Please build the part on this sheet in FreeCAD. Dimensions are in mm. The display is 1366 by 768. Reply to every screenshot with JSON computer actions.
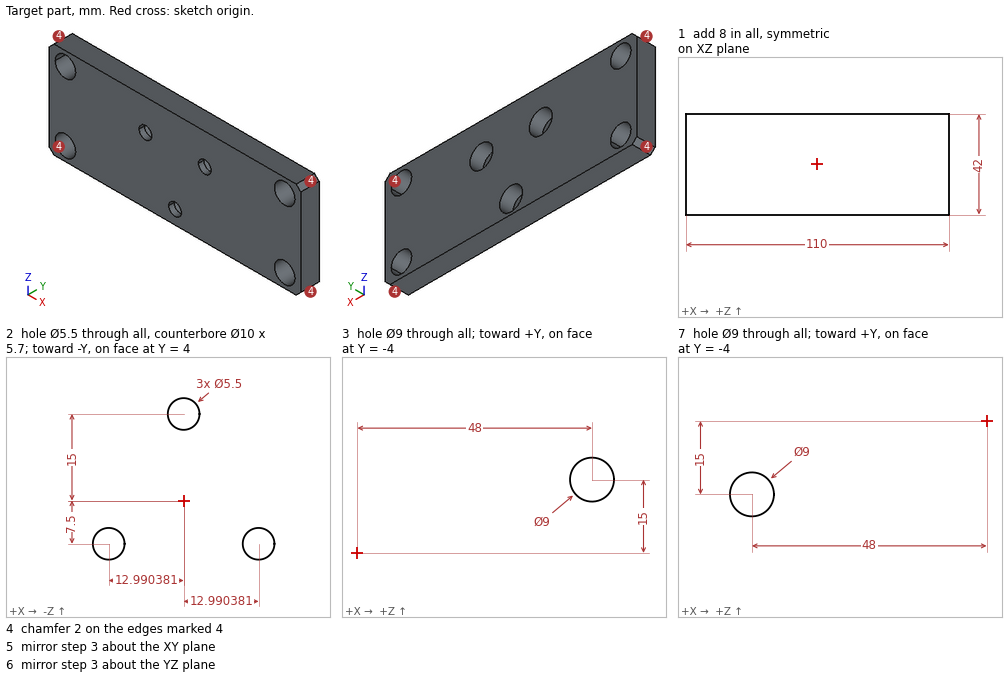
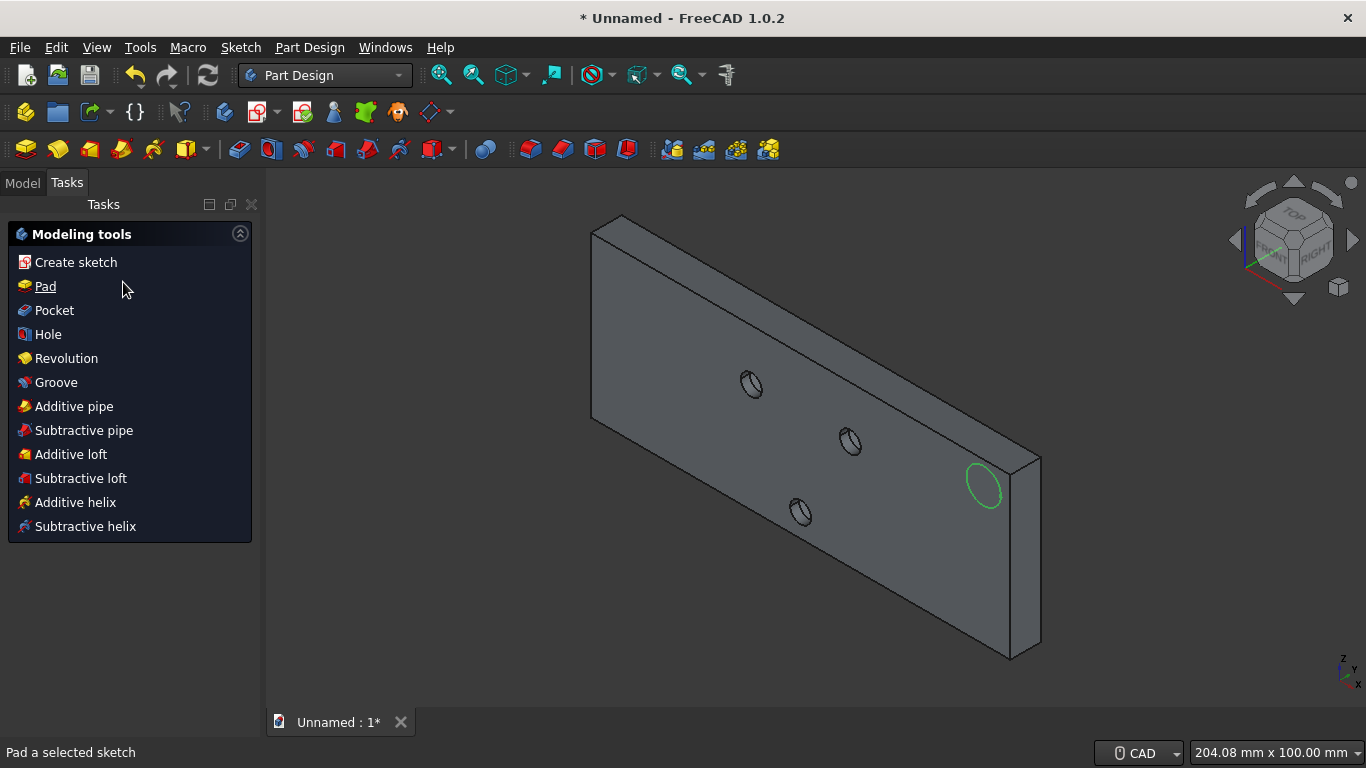
{"action": "left_click", "coordinate": [272, 150]}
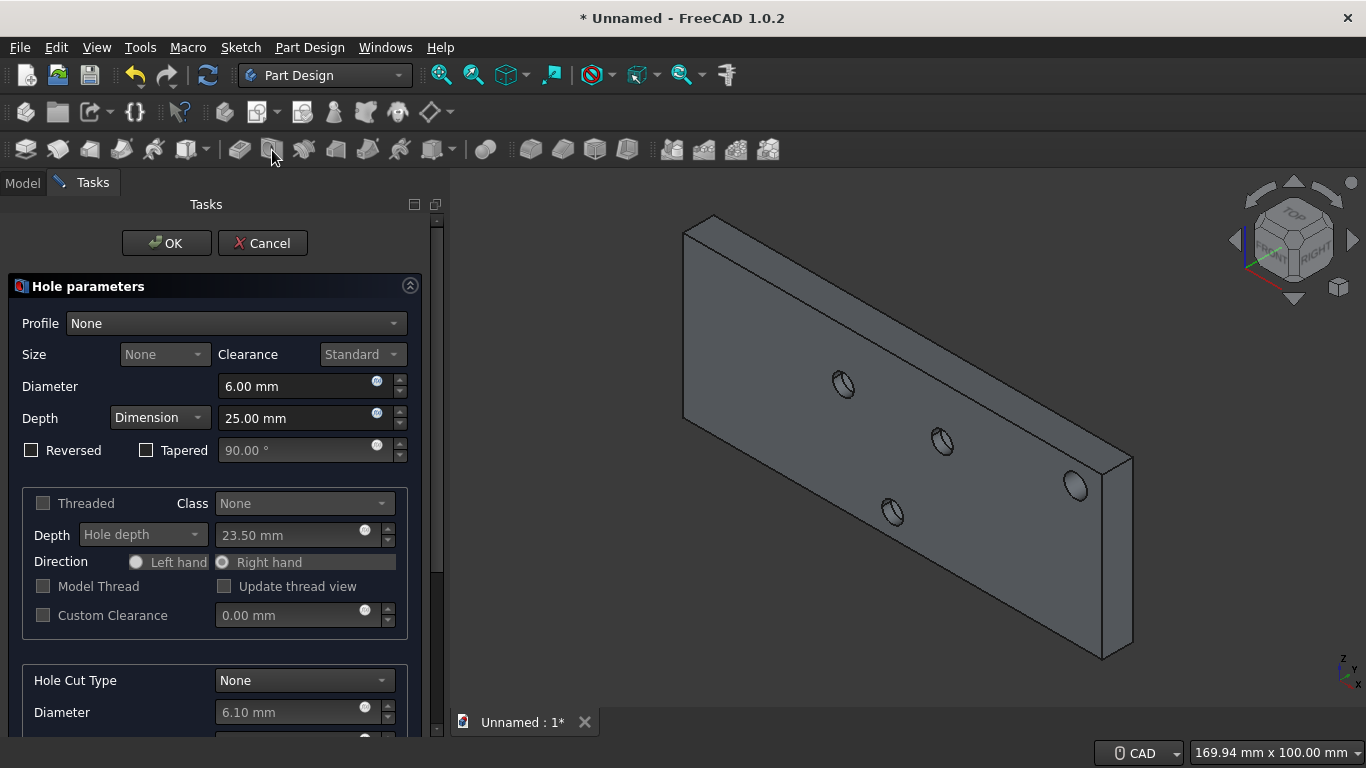
{"action": "triple_click", "coordinate": [305, 386]}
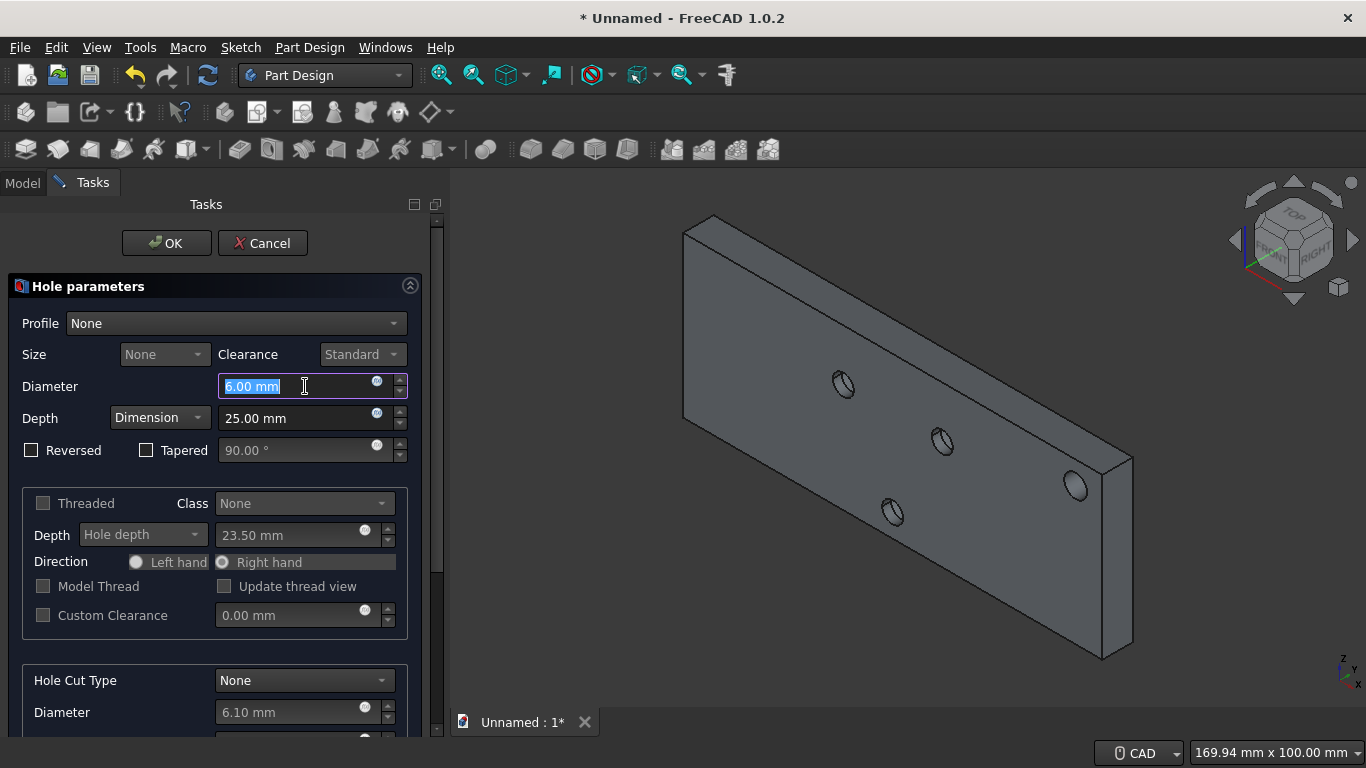
{"action": "type", "text": "9"}
{"action": "key", "text": "Tab"}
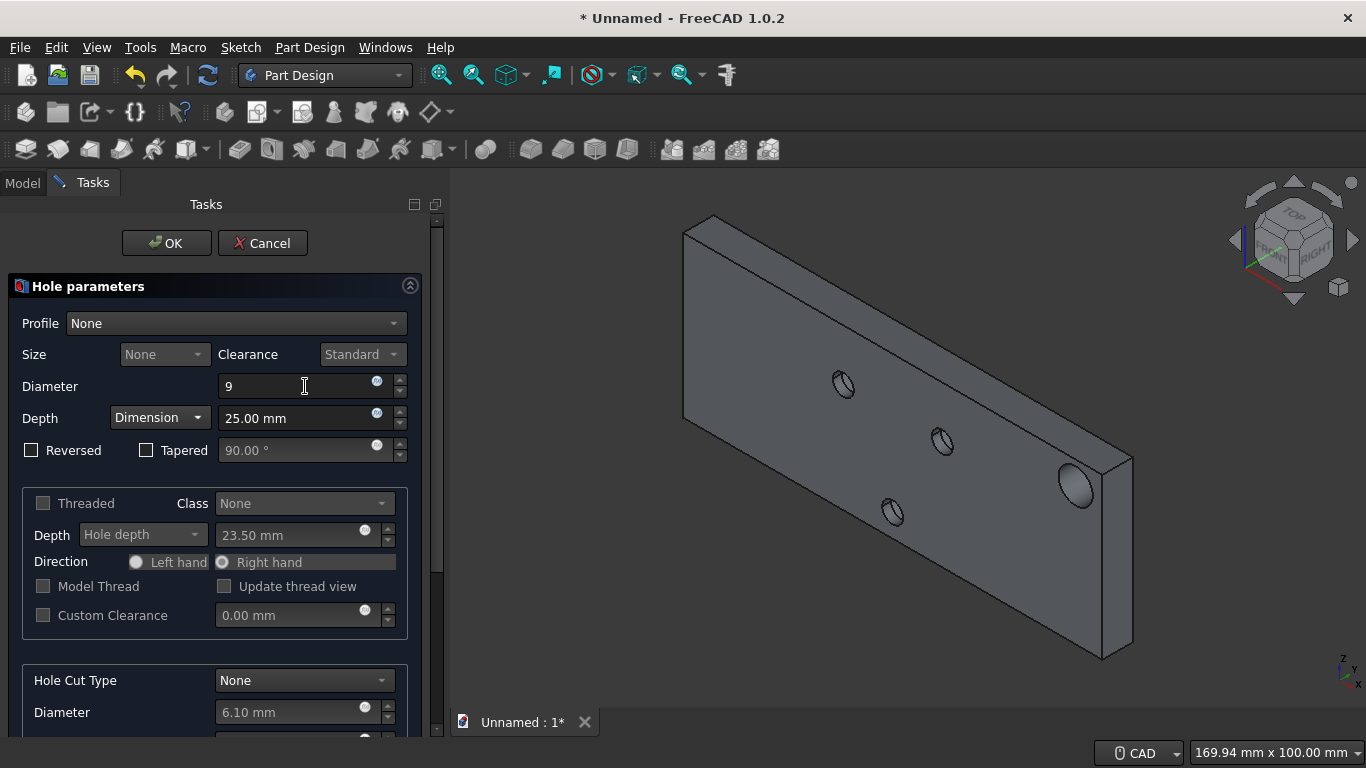
{"action": "left_click", "coordinate": [161, 418]}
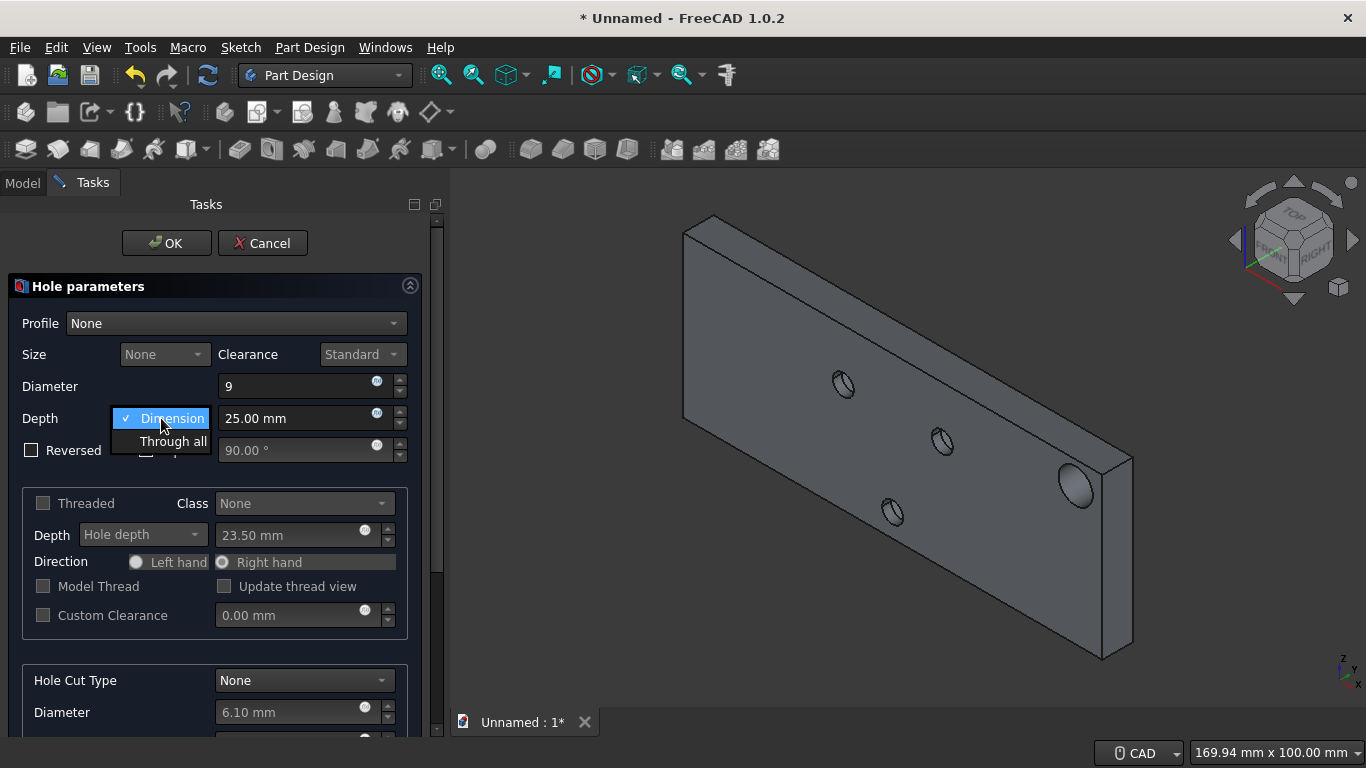
{"action": "left_click", "coordinate": [160, 442]}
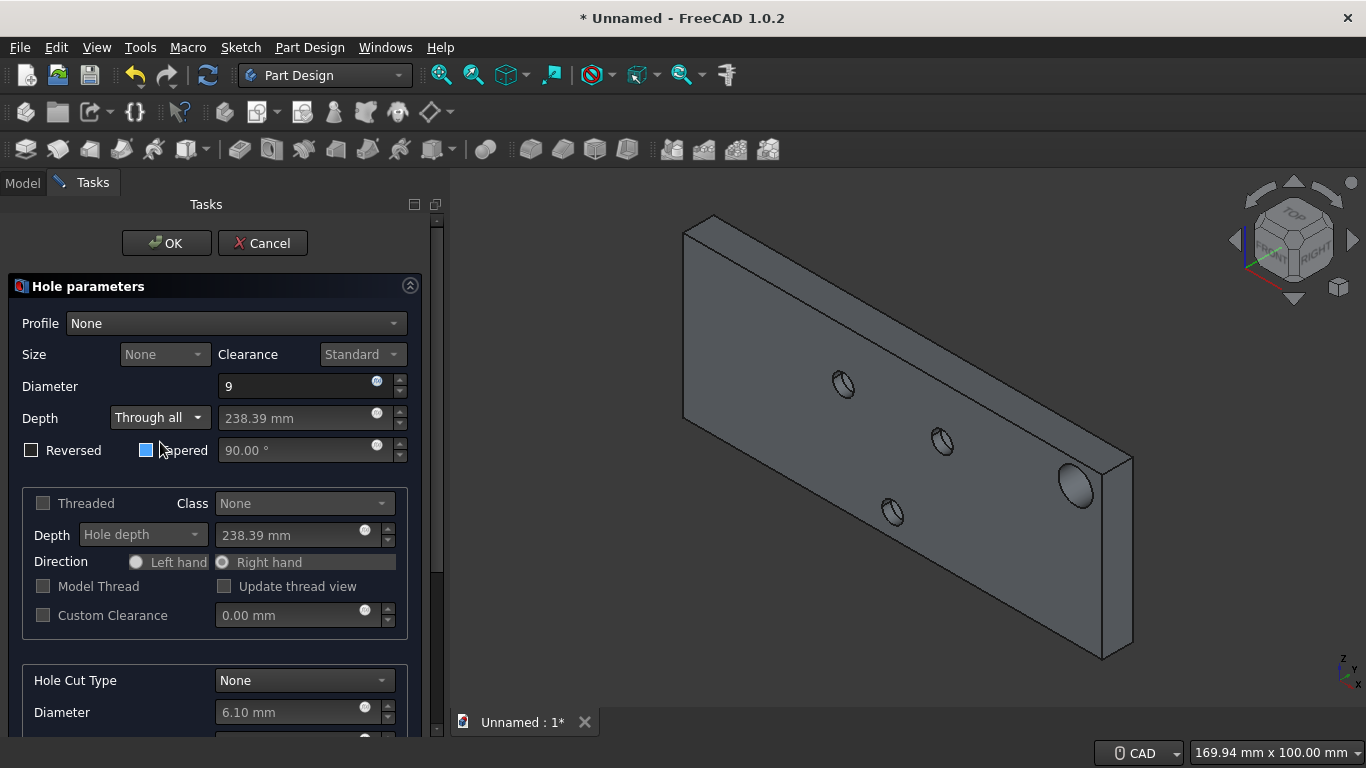
{"action": "left_click", "coordinate": [167, 243]}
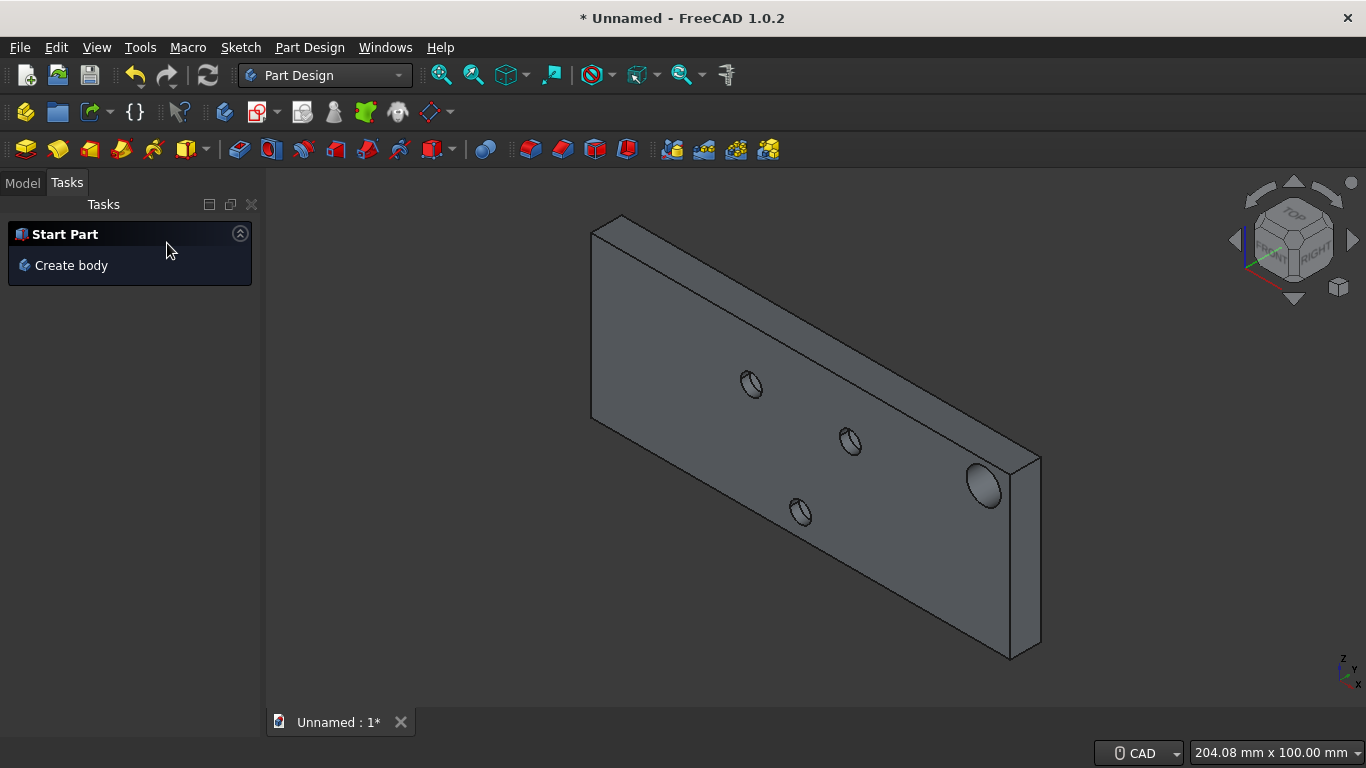
{"action": "left_click", "coordinate": [1026, 465]}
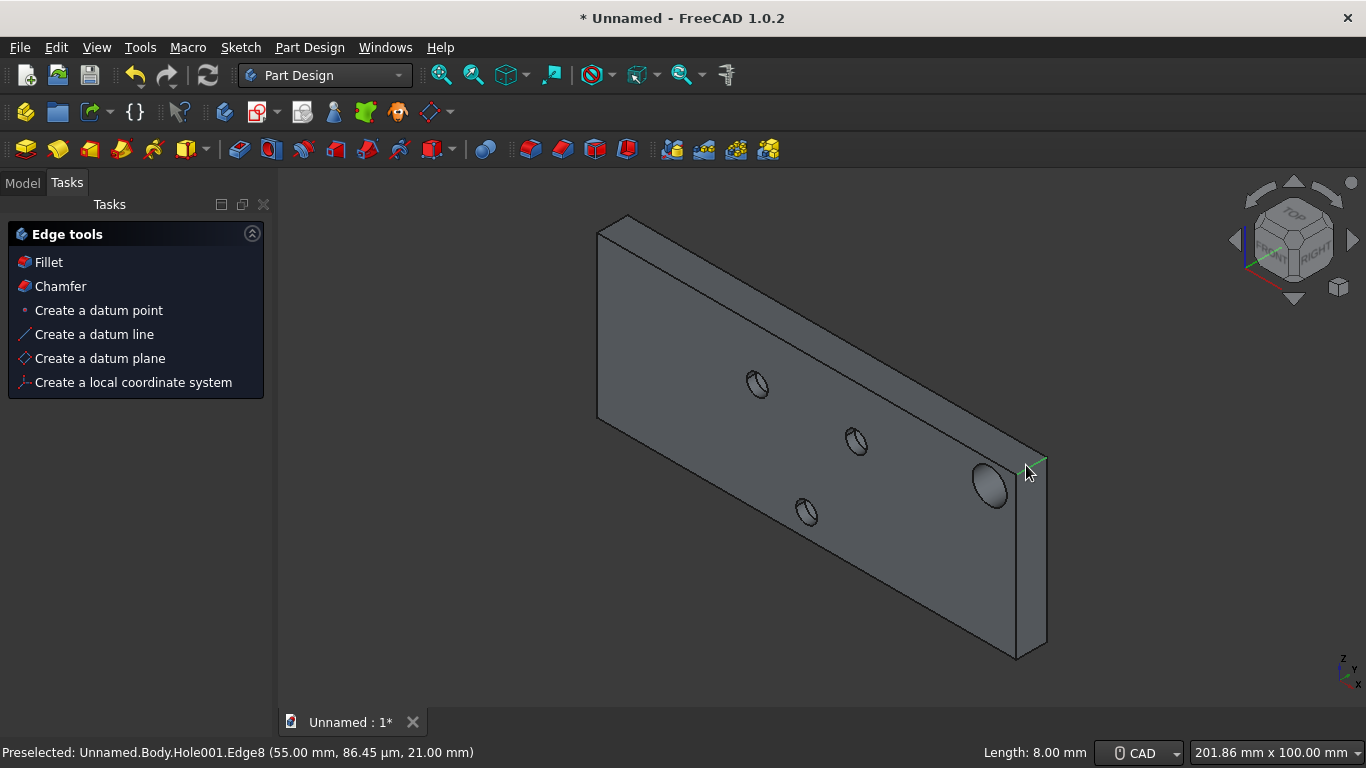
{"action": "key", "text": "2"}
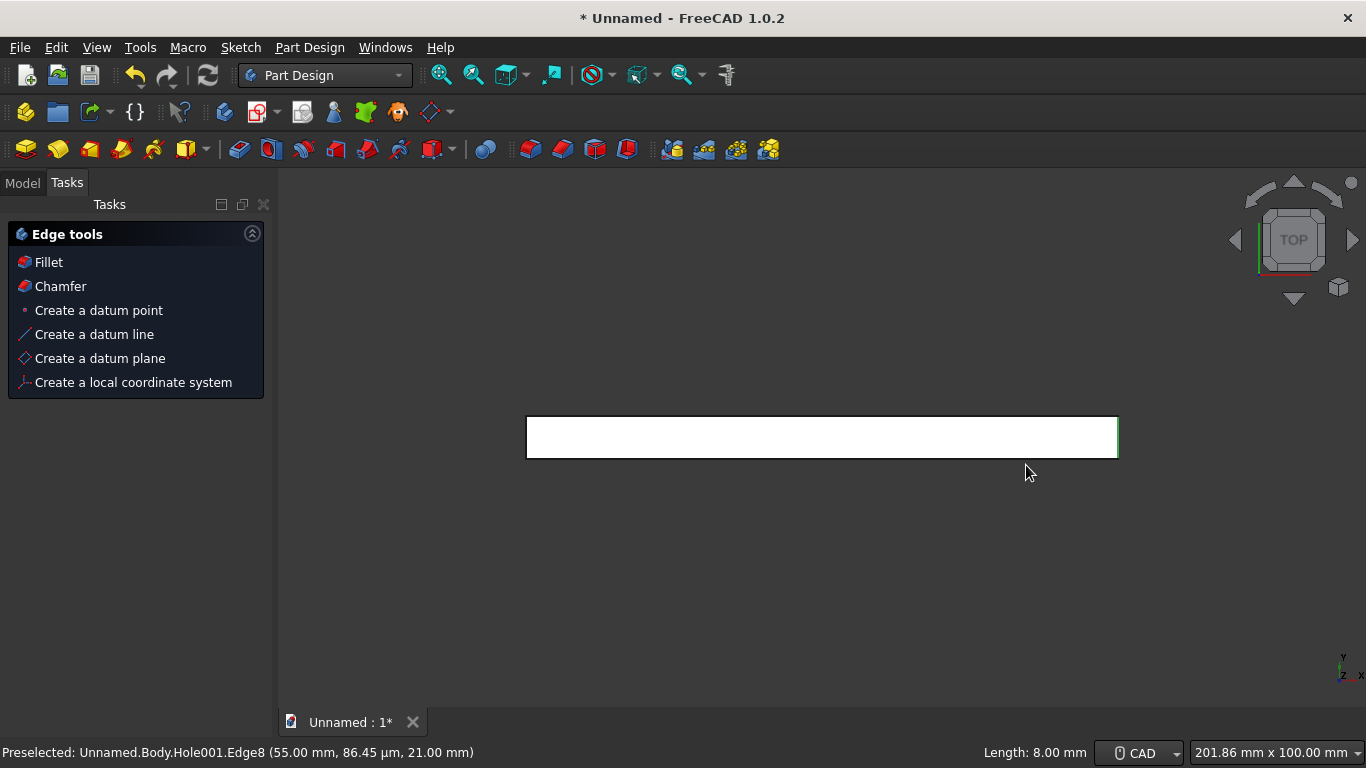
{"action": "left_click", "coordinate": [526, 436], "text": "ctrl"}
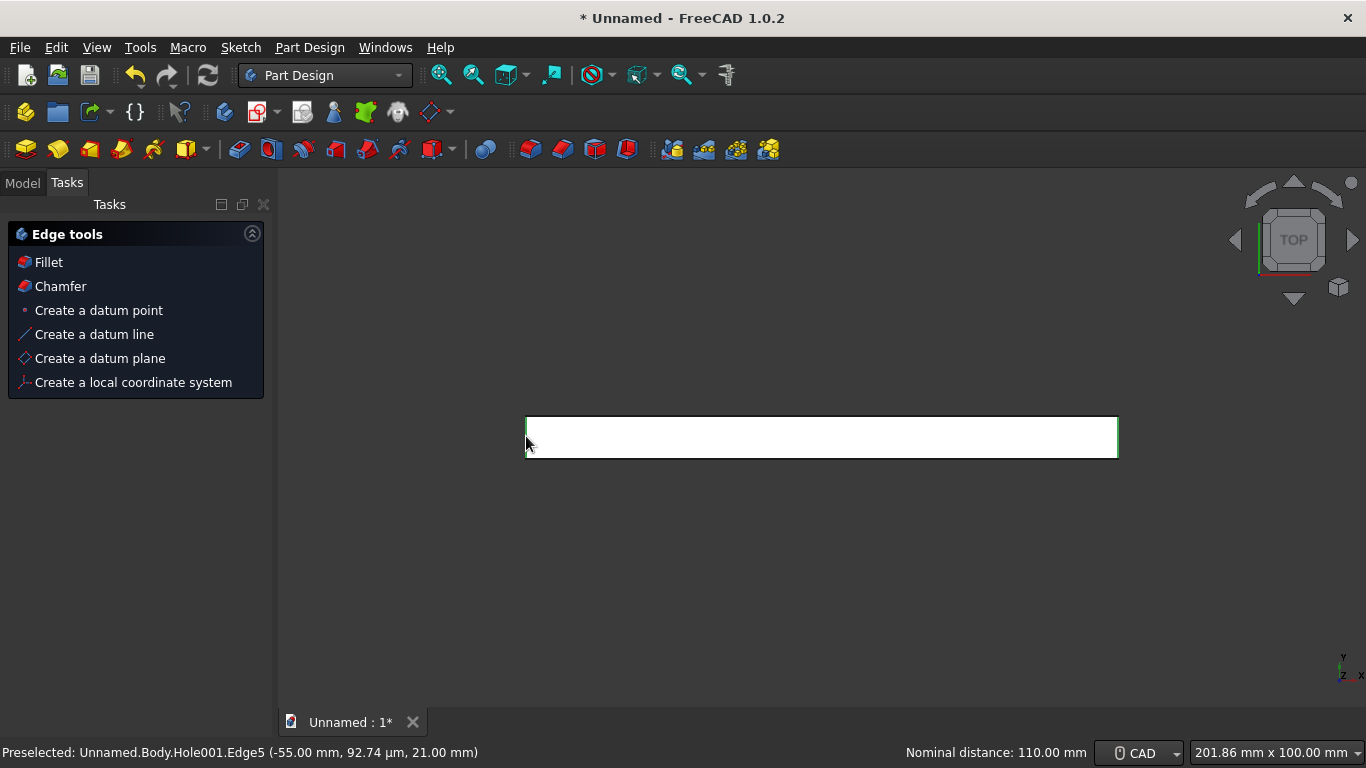
{"action": "key", "text": "0"}